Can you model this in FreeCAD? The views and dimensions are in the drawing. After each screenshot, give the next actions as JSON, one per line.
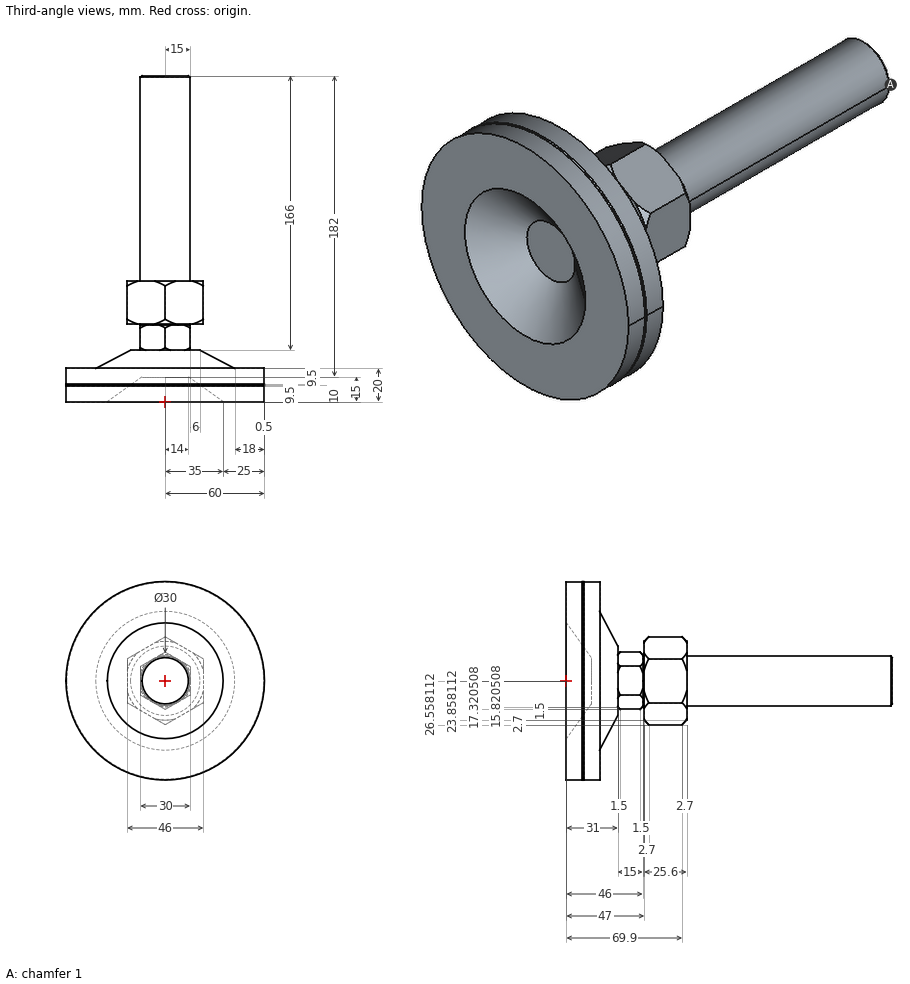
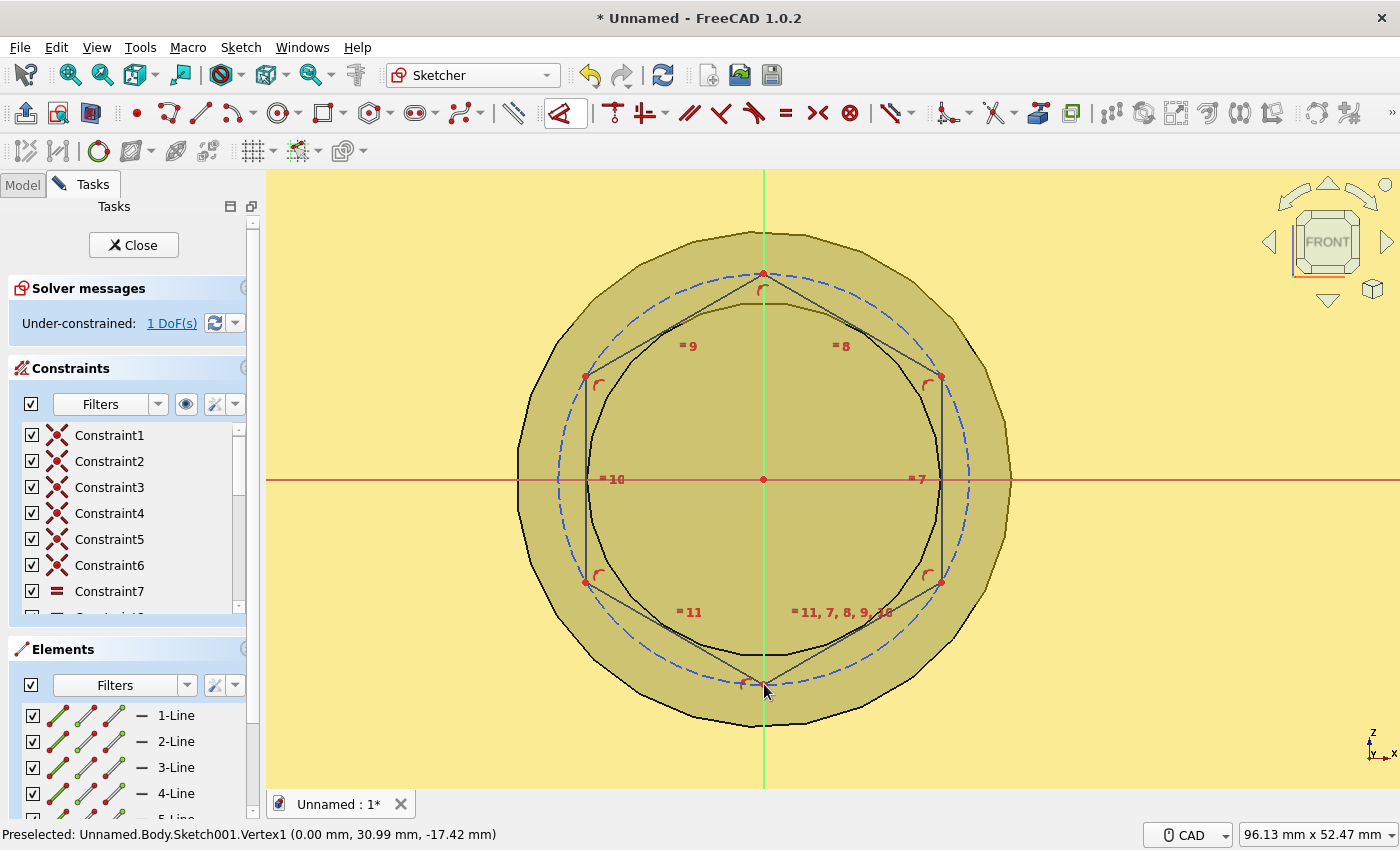
{"action": "left_click", "coordinate": [586, 377]}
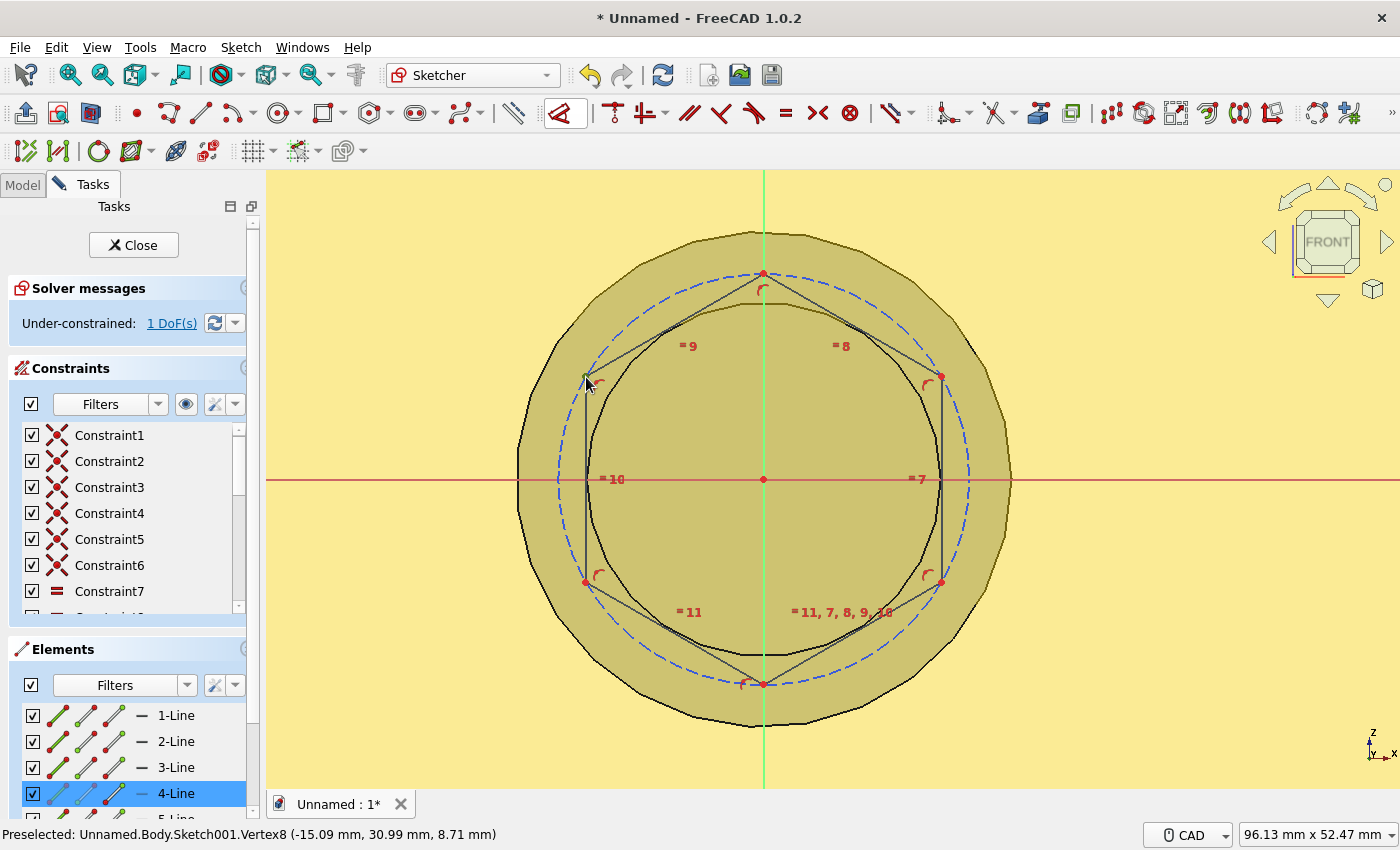
{"action": "left_click", "coordinate": [942, 582]}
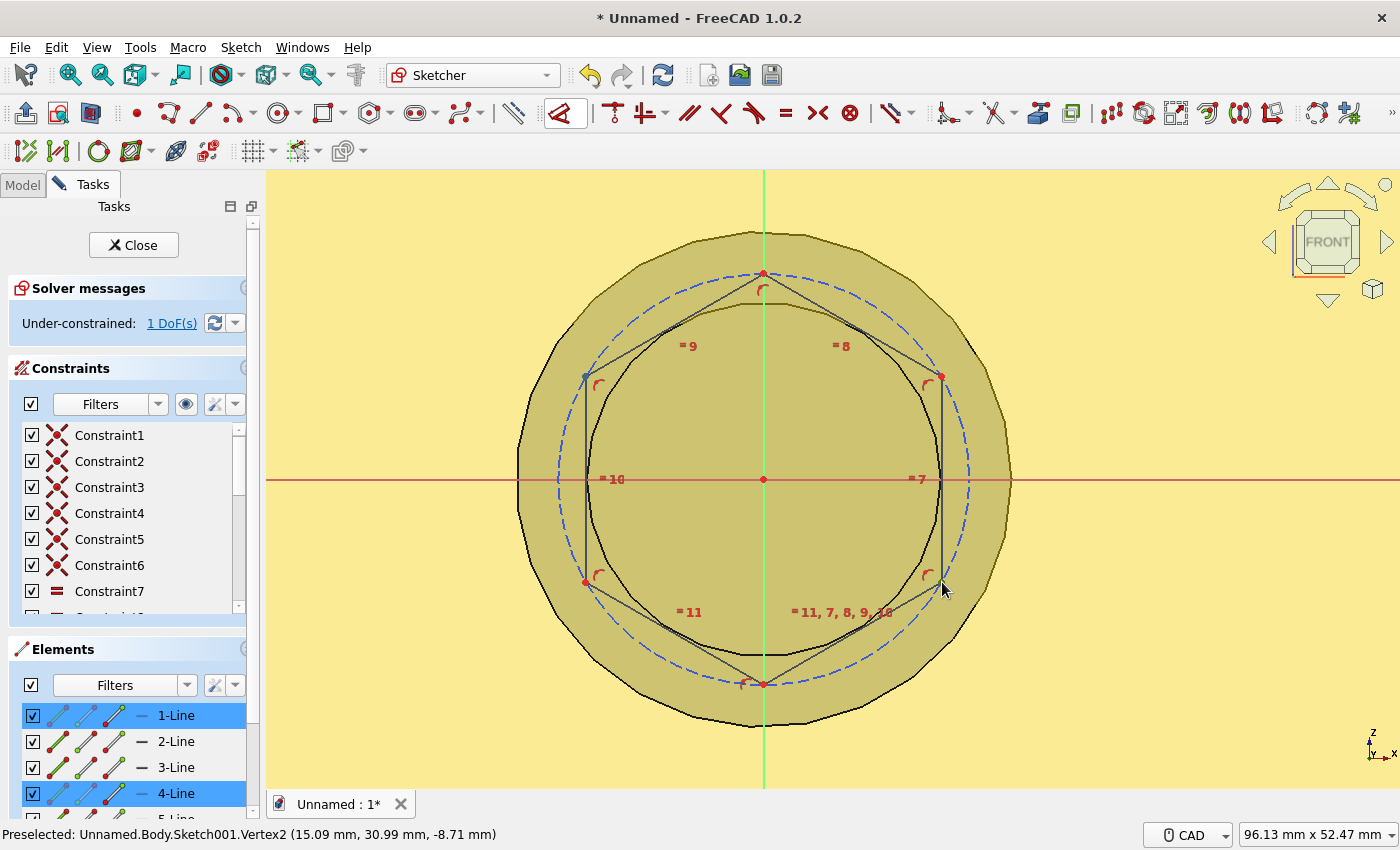
{"action": "left_click", "coordinate": [582, 114]}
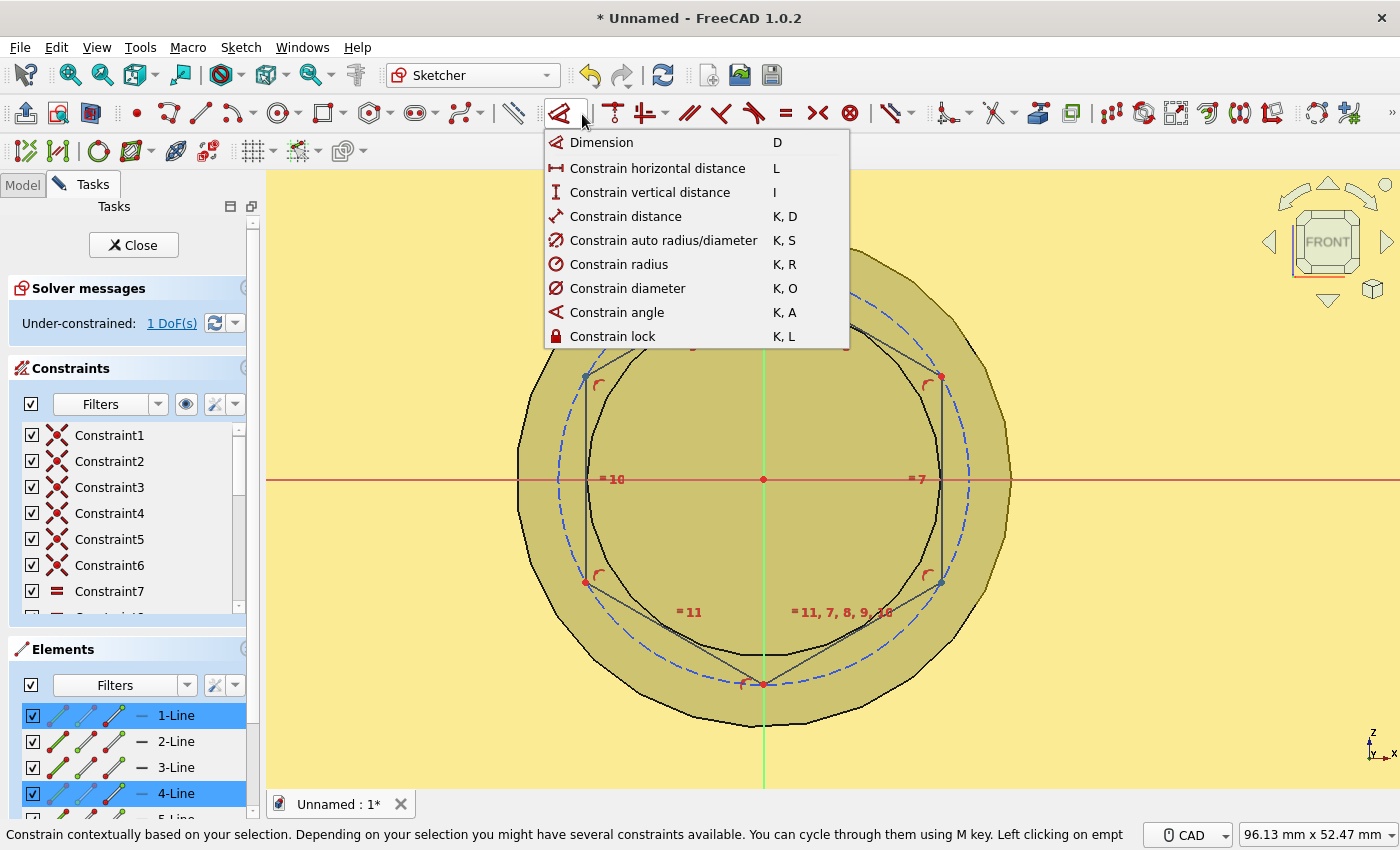
{"action": "left_click", "coordinate": [697, 168]}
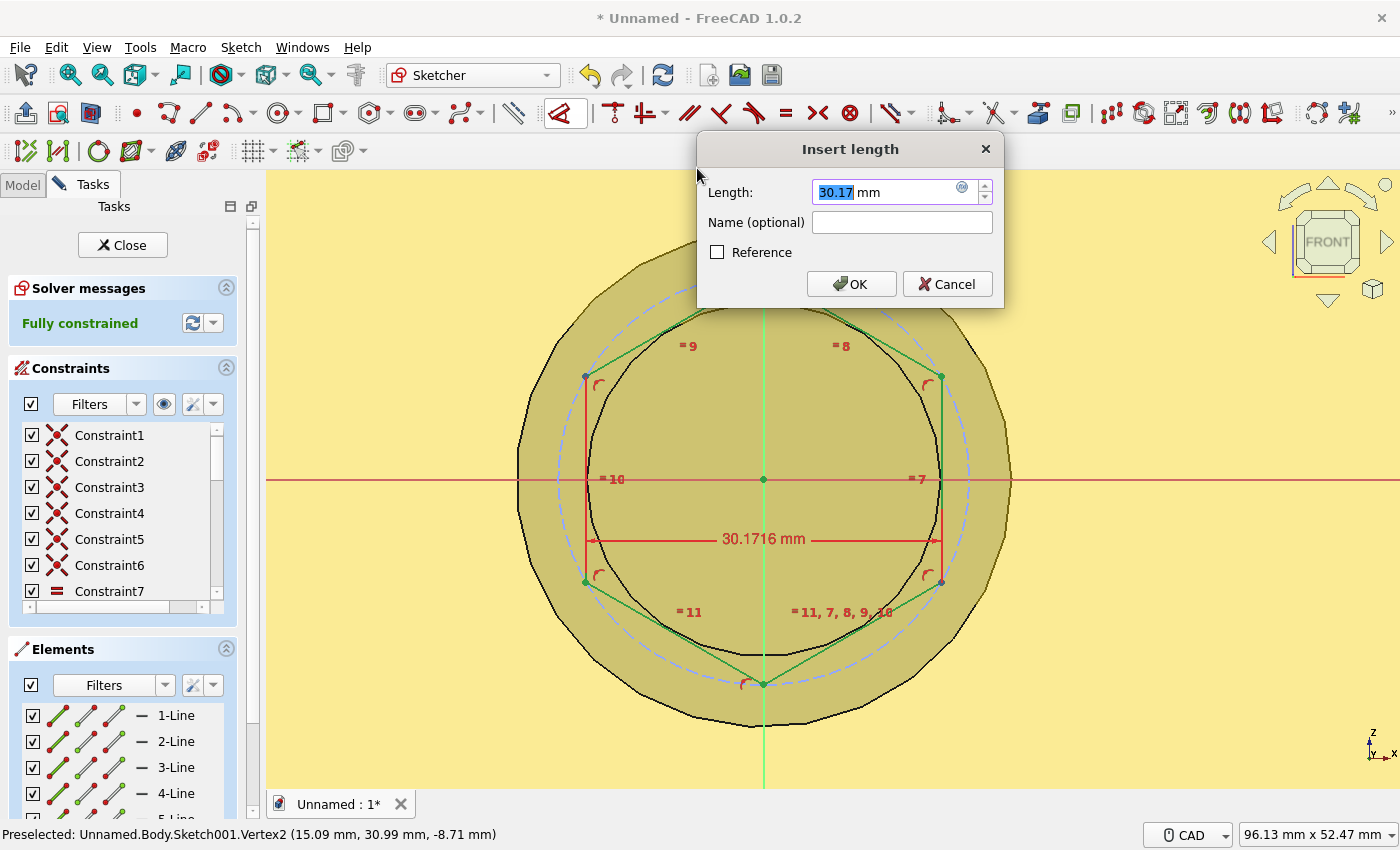
{"action": "type", "text": "30"}
{"action": "key", "text": "Return"}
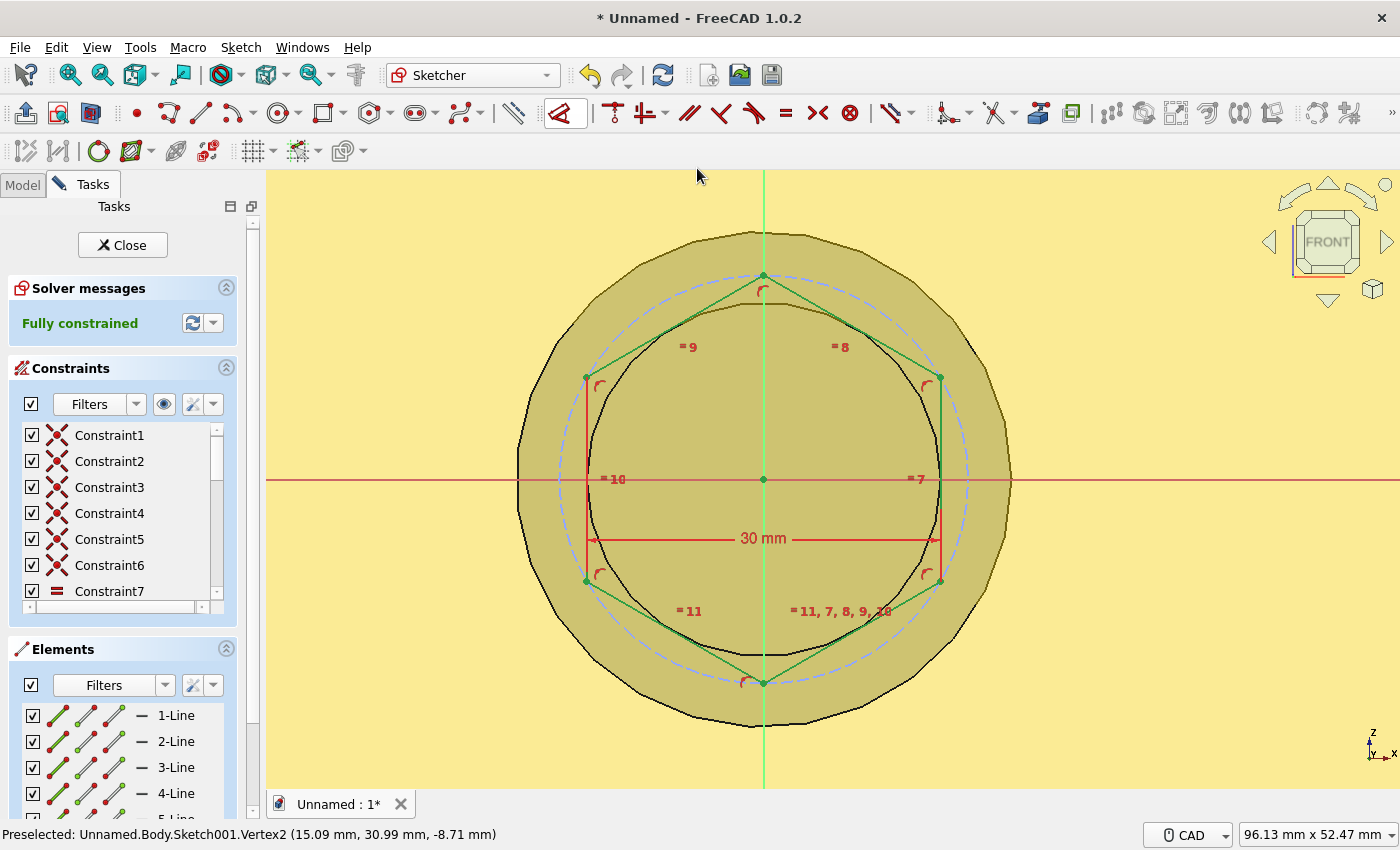
{"action": "left_click", "coordinate": [123, 245]}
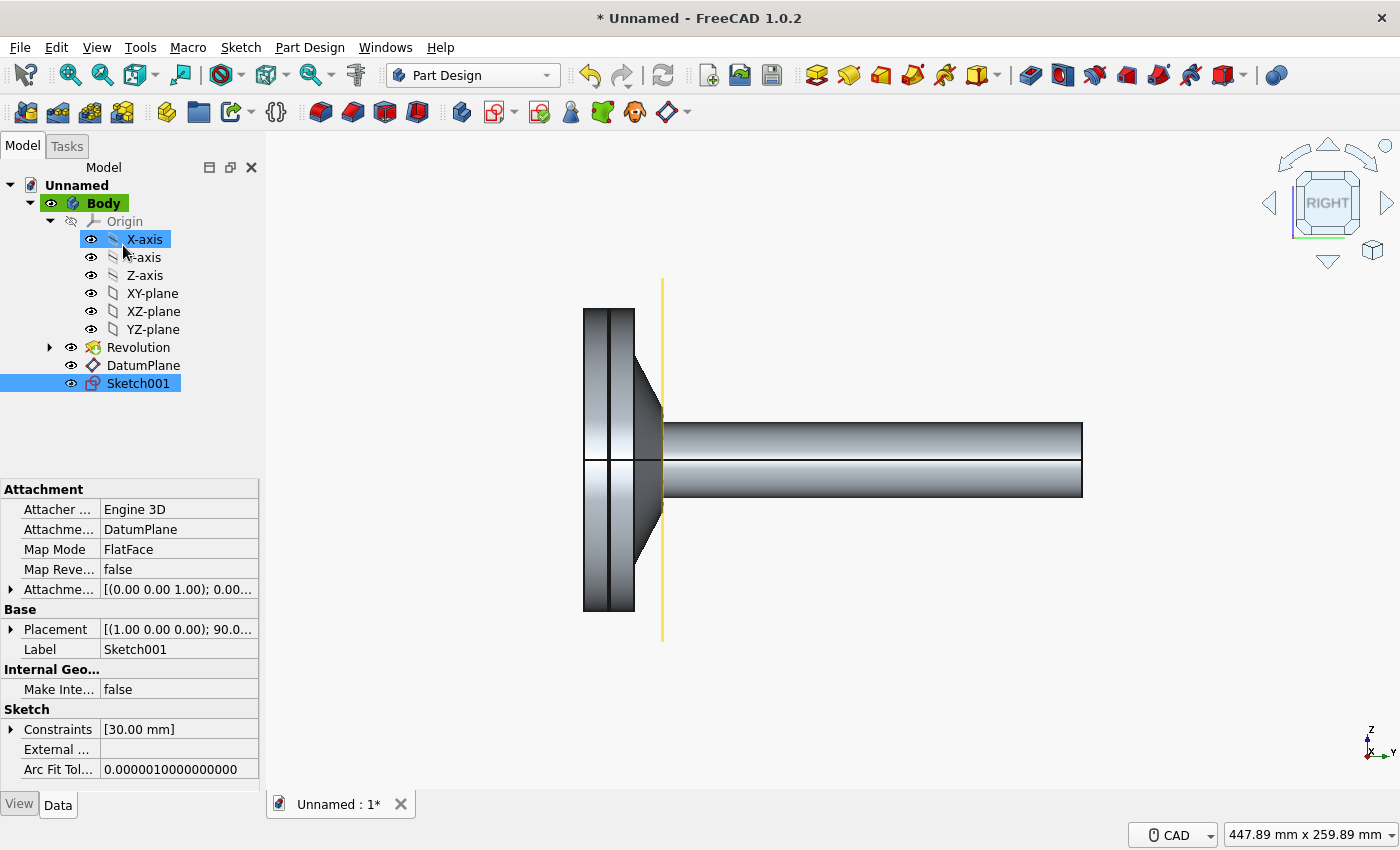
{"action": "left_click", "coordinate": [818, 76]}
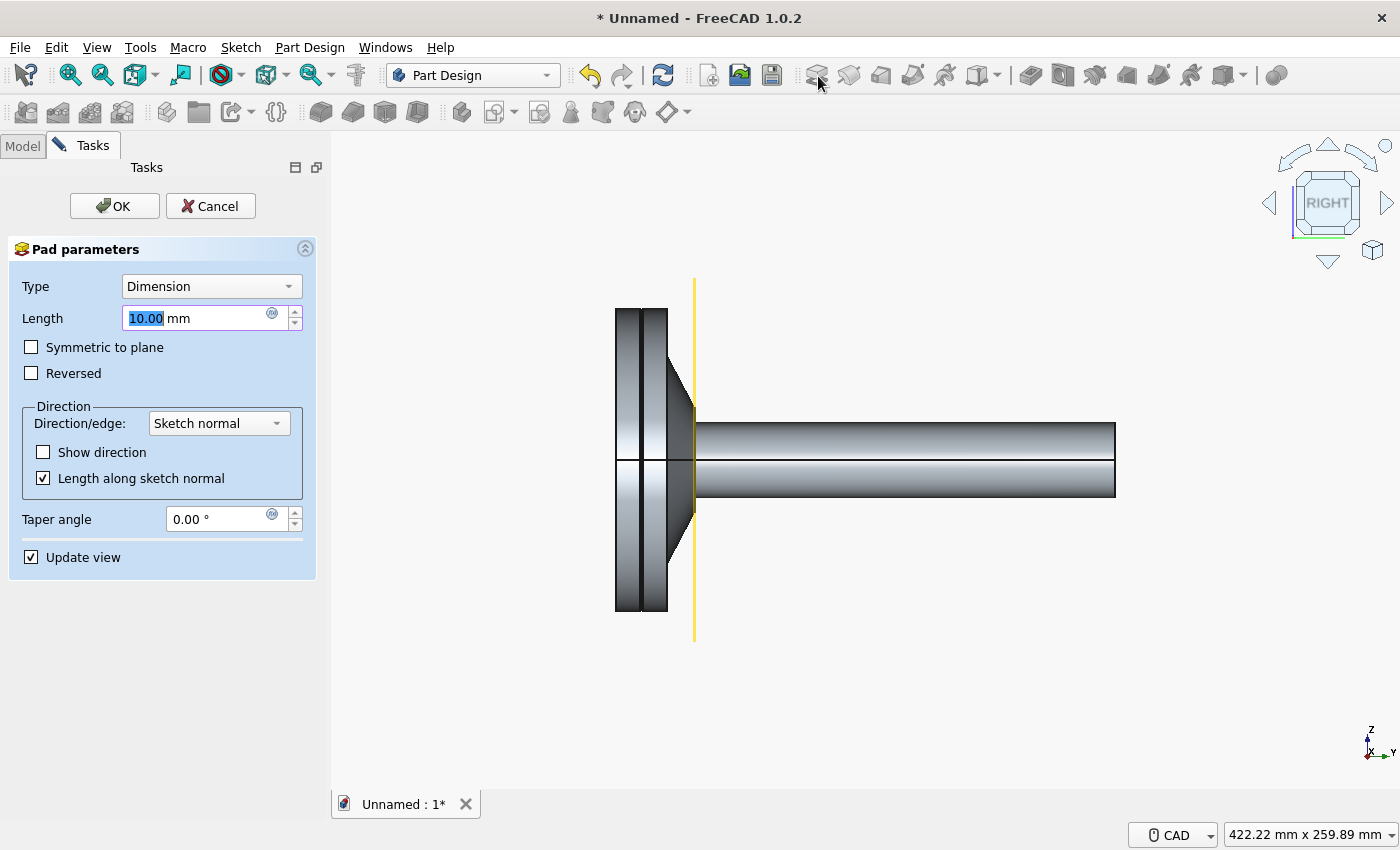
{"action": "type", "text": "15"}
{"action": "key", "text": "Tab"}